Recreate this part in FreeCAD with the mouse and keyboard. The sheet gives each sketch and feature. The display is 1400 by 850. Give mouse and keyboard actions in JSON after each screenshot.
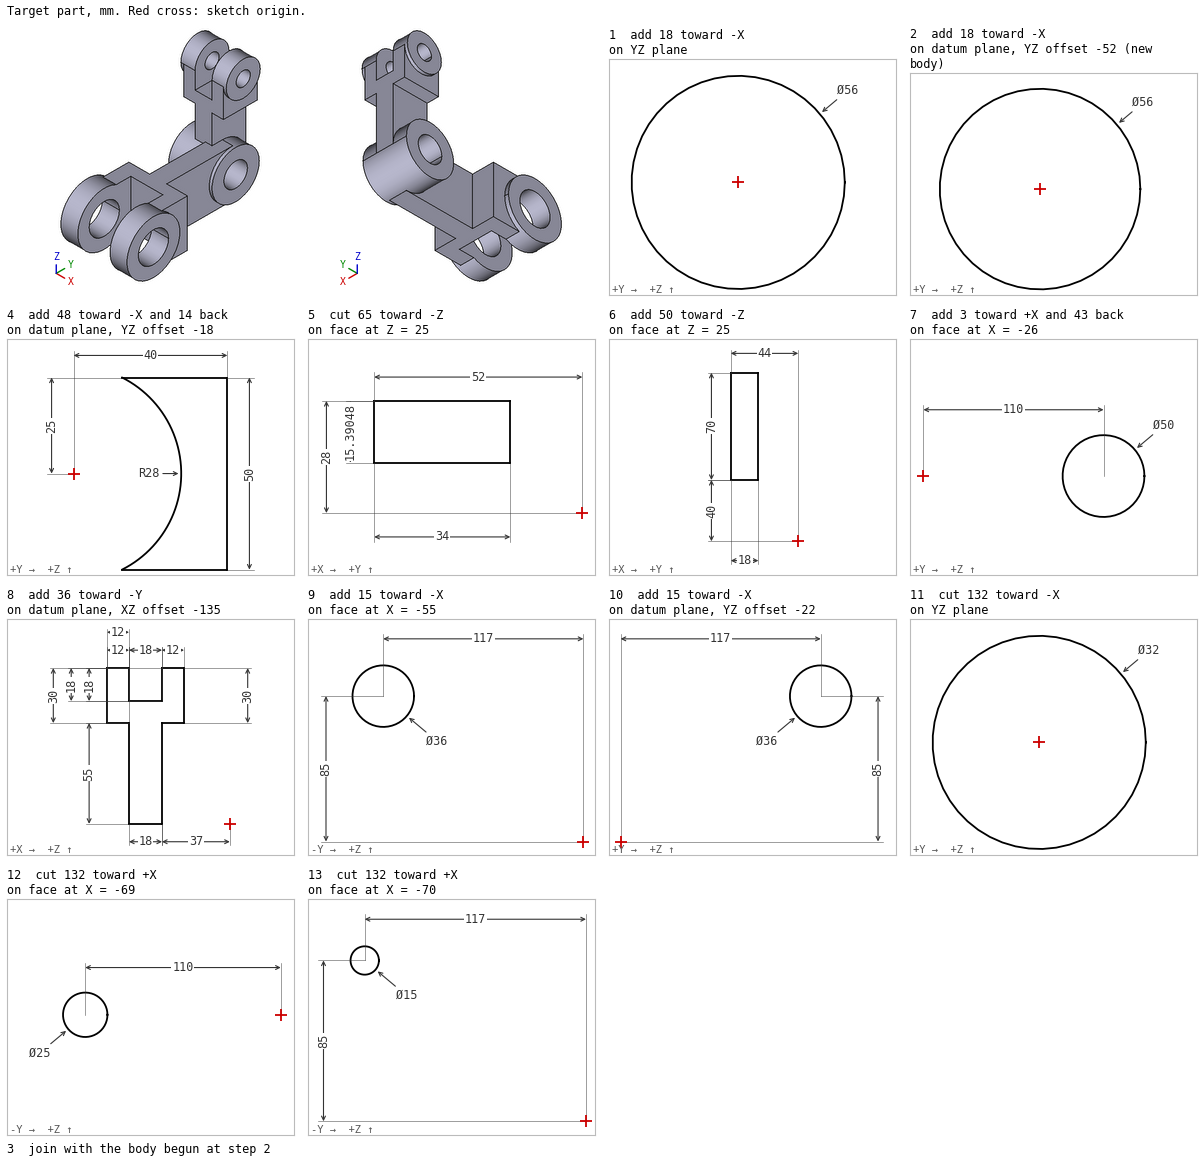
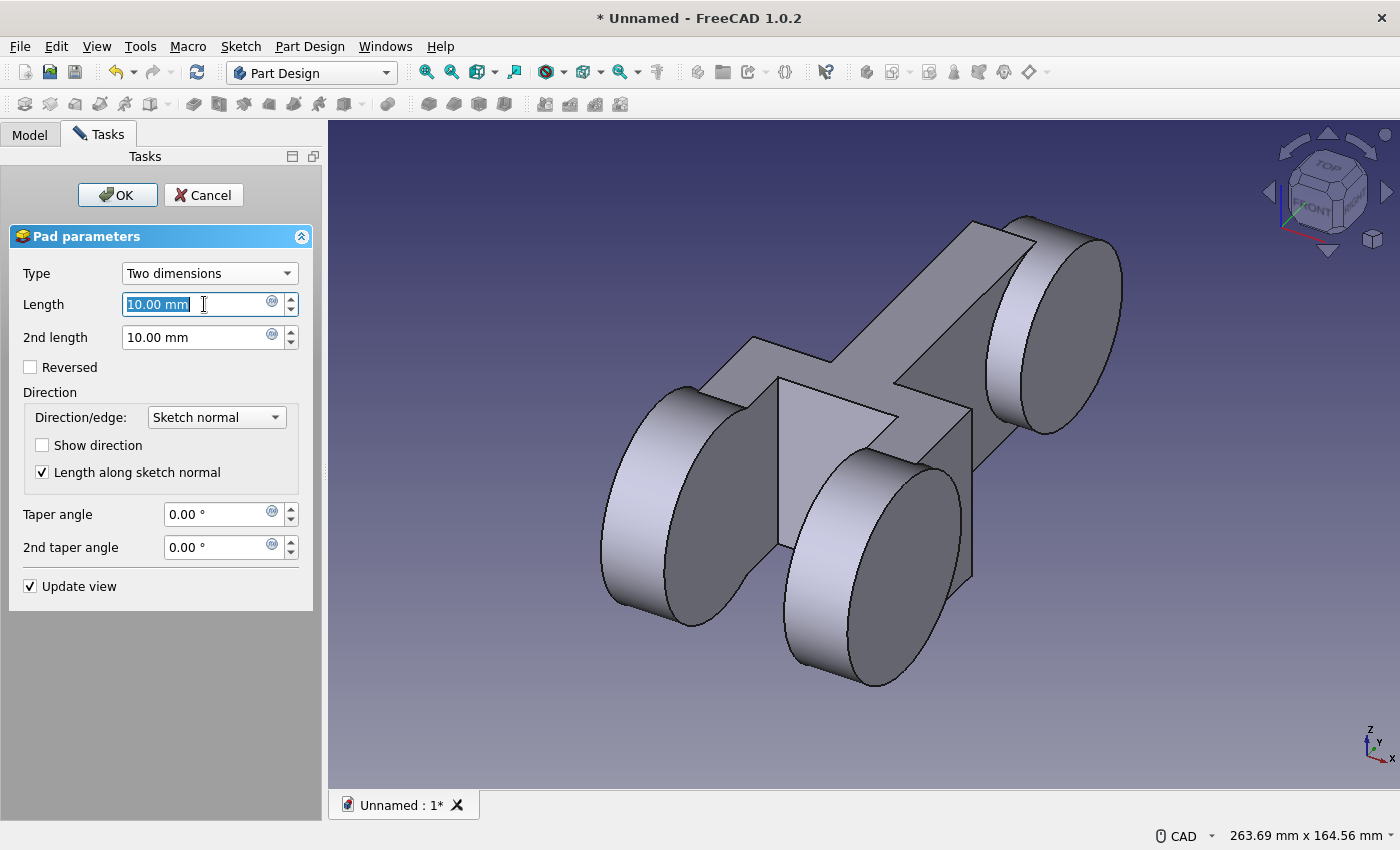
{"action": "type", "text": "3"}
{"action": "key", "text": "Tab"}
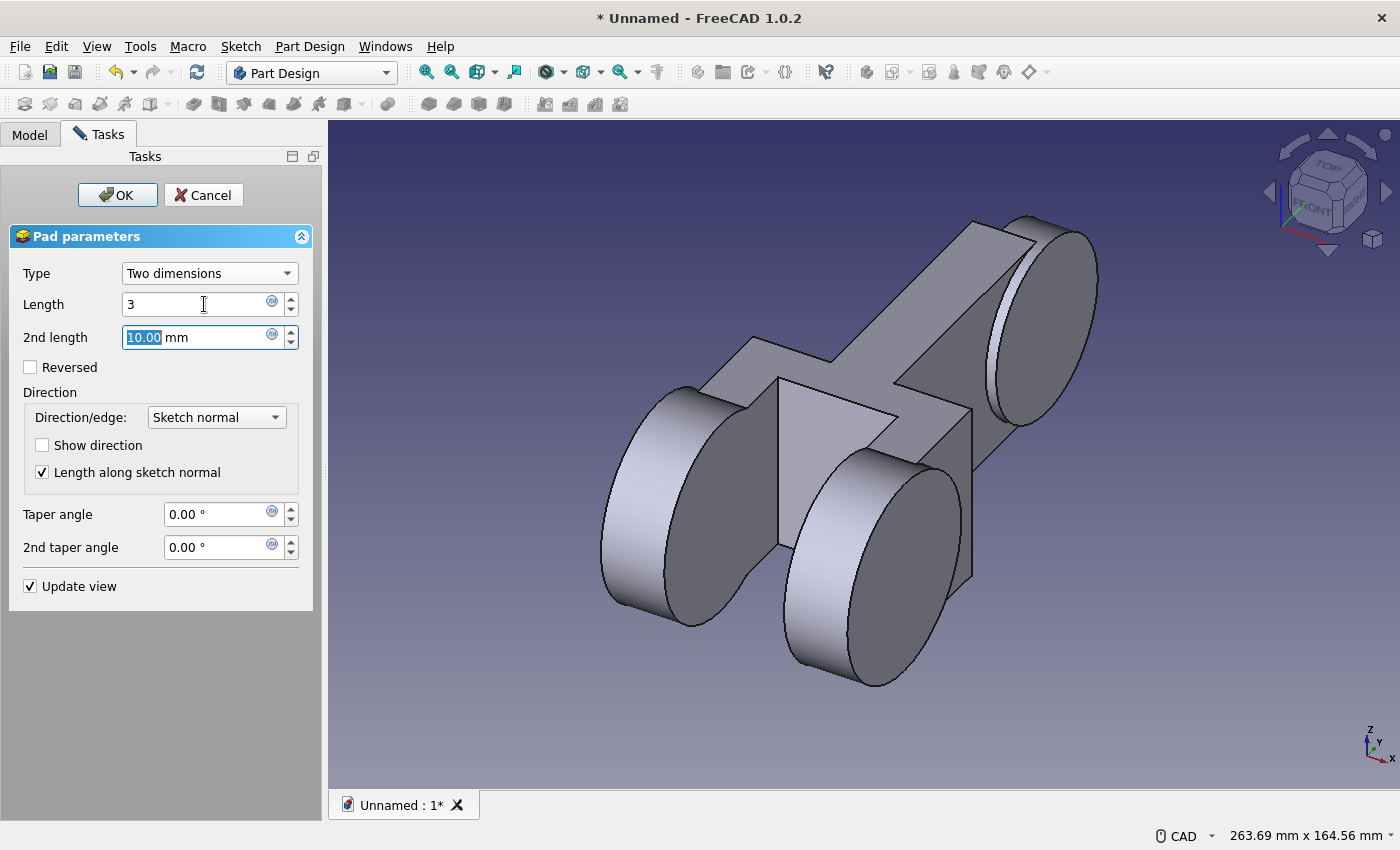
{"action": "type", "text": "43"}
{"action": "key", "text": "Tab"}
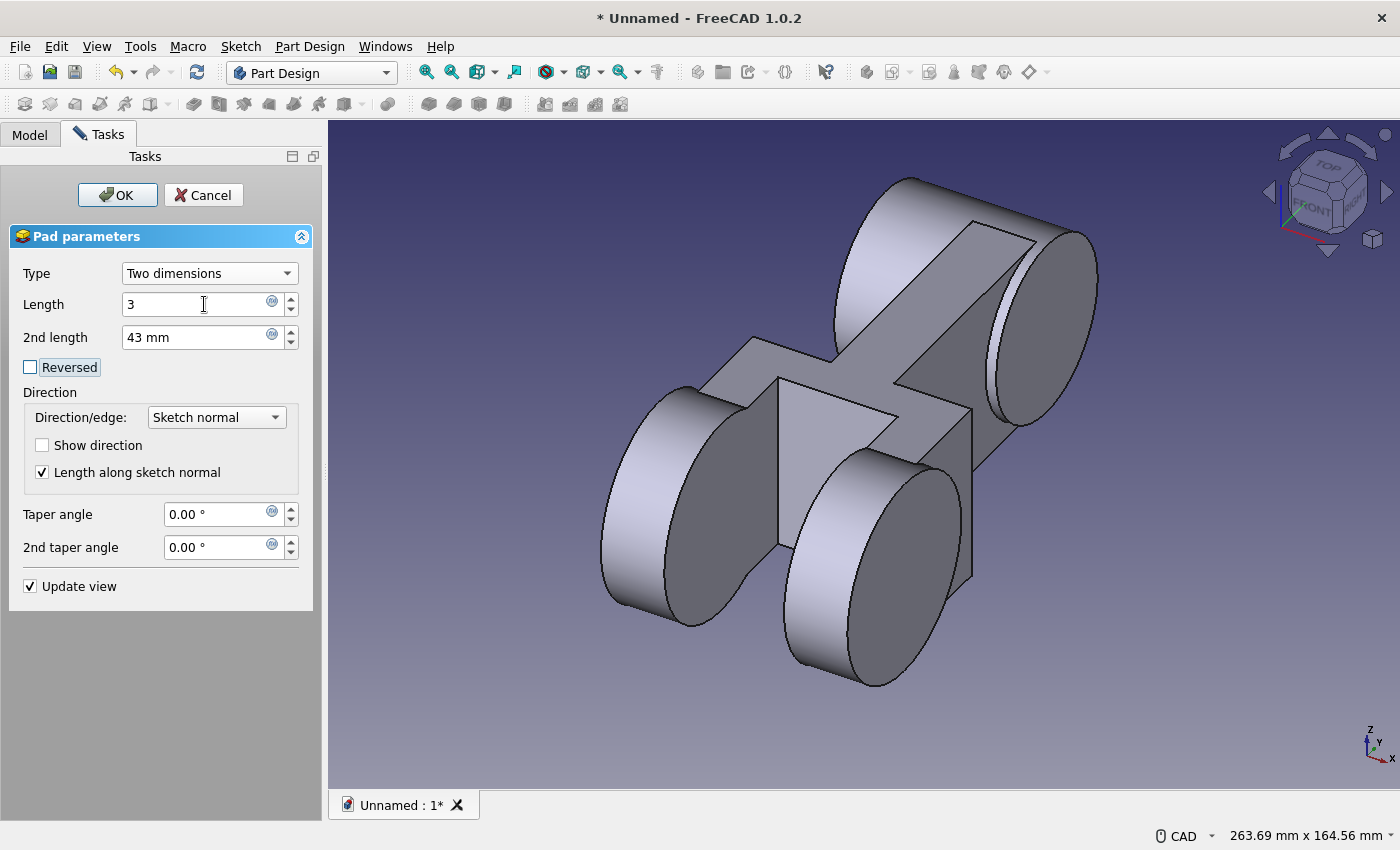
{"action": "left_click", "coordinate": [118, 195]}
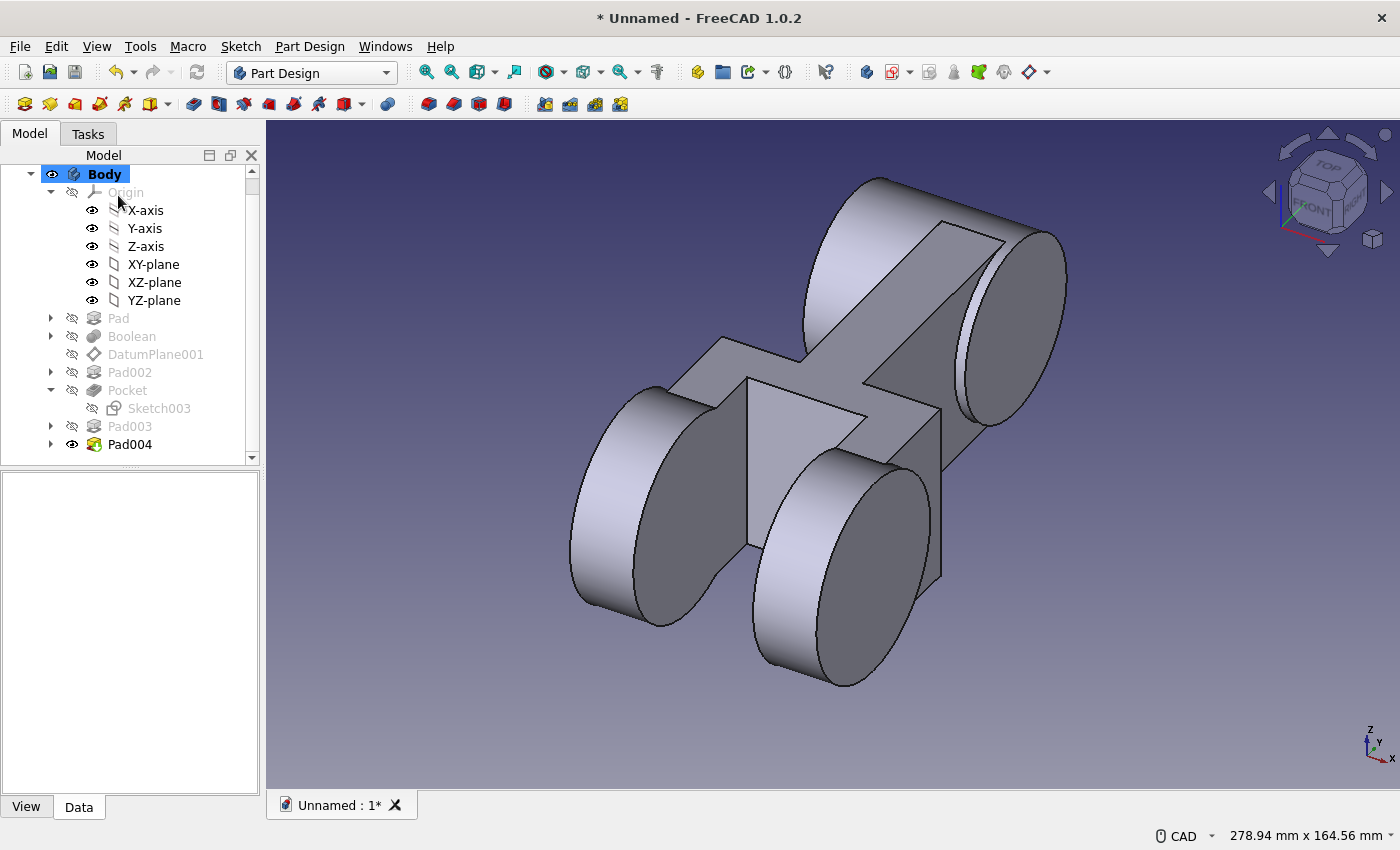
{"action": "left_click", "coordinate": [137, 282]}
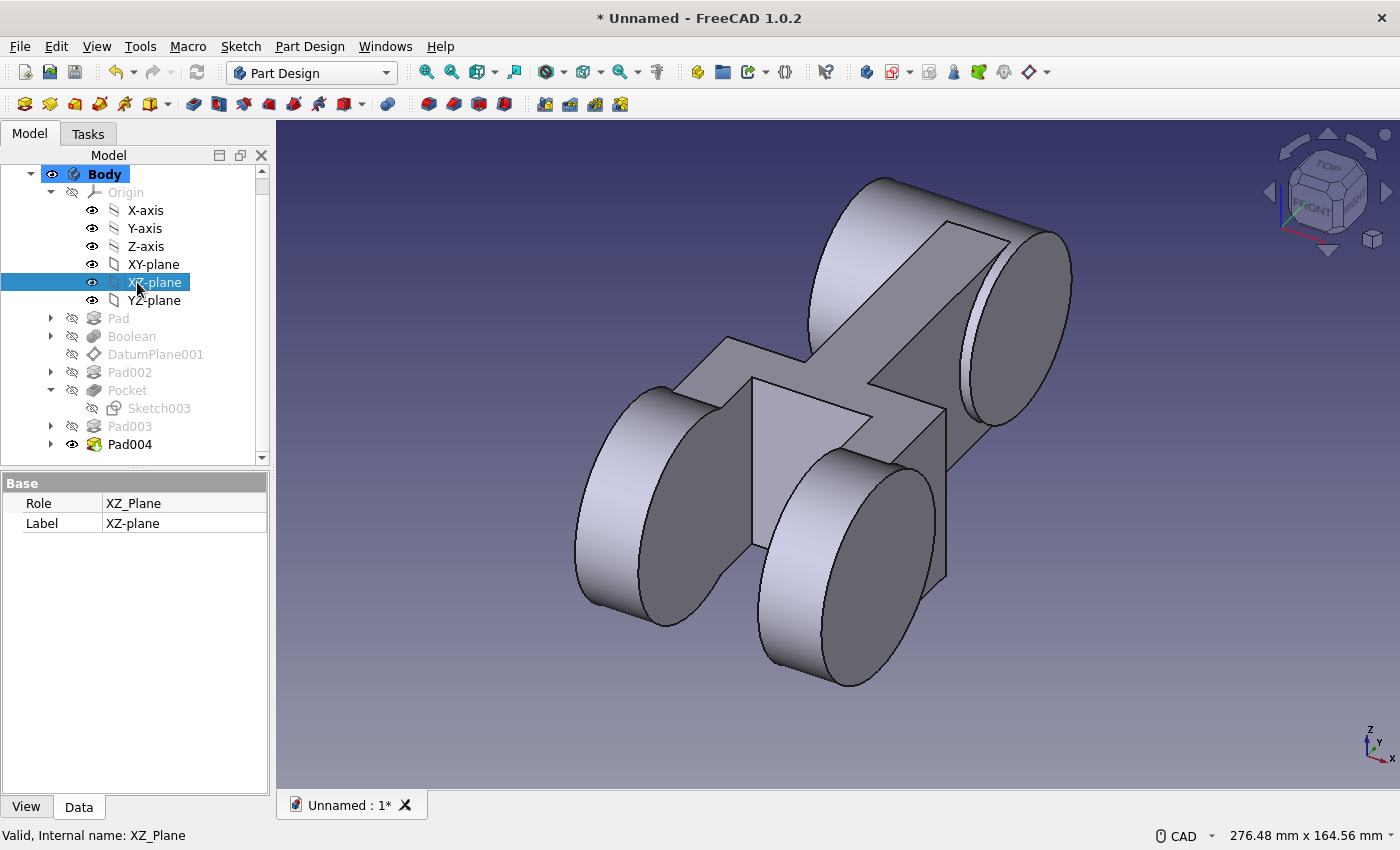
{"action": "left_click", "coordinate": [1028, 72]}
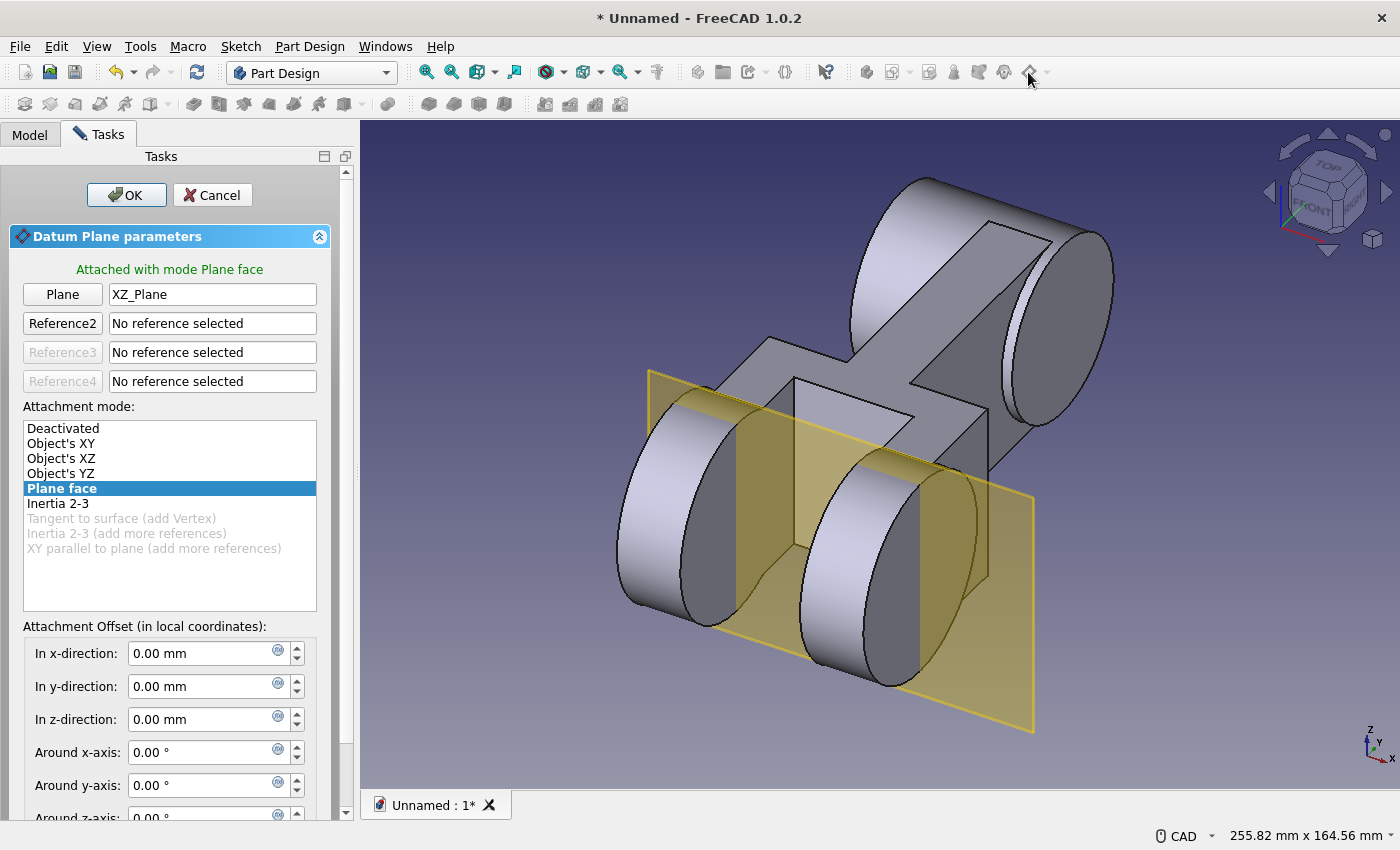
{"action": "triple_click", "coordinate": [210, 720]}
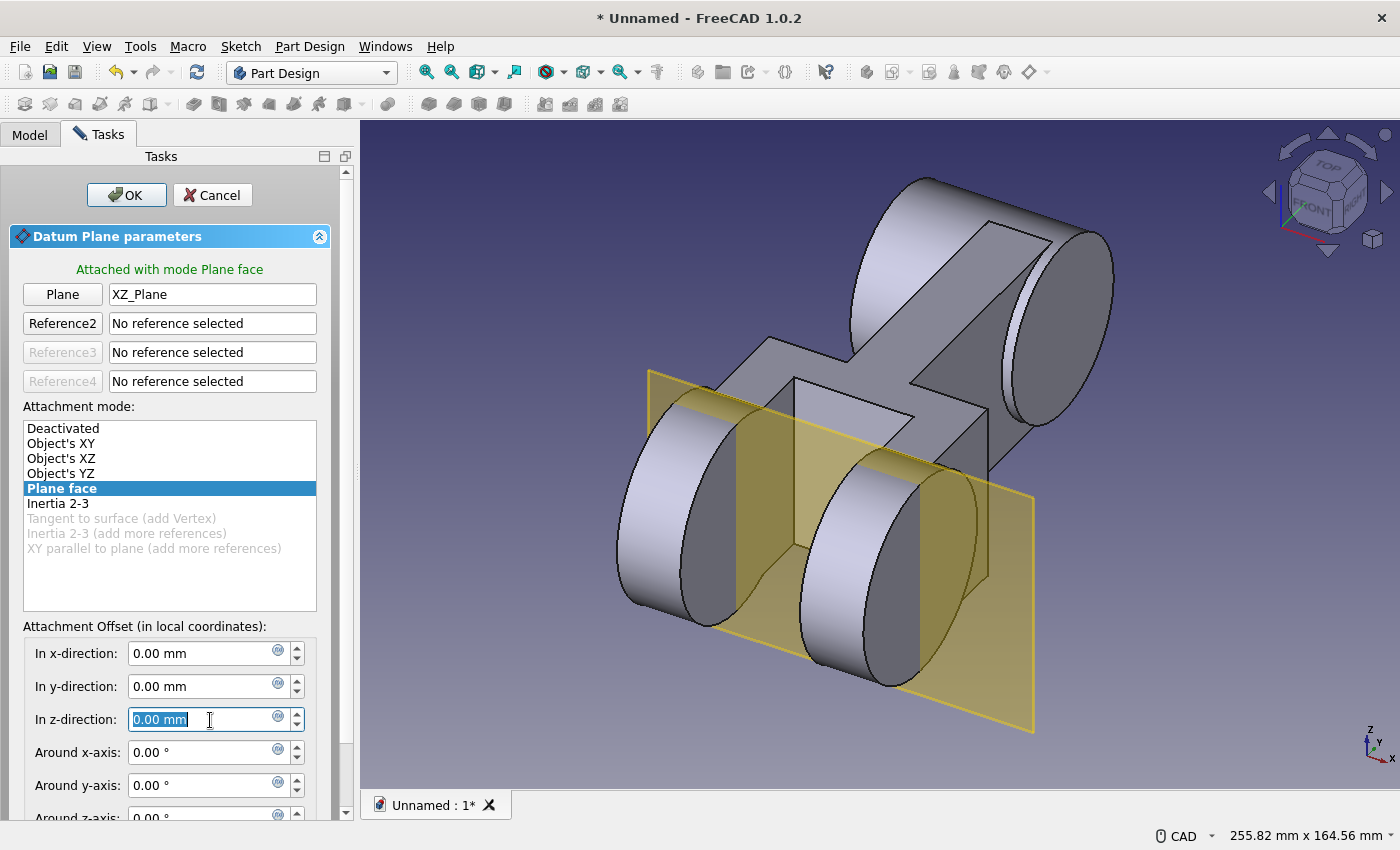
{"action": "type", "text": "-135"}
{"action": "key", "text": "Tab"}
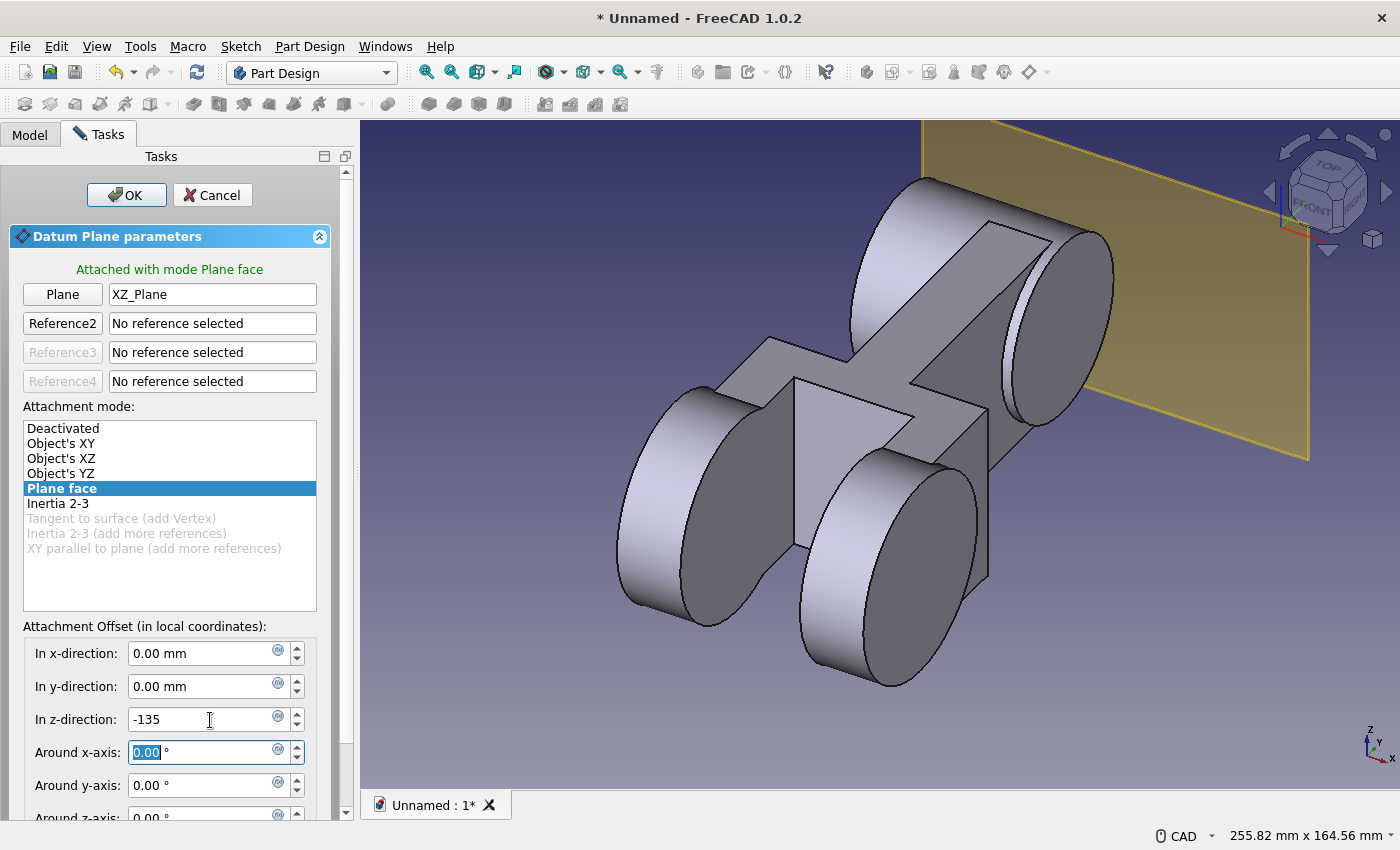
{"action": "left_click", "coordinate": [127, 195]}